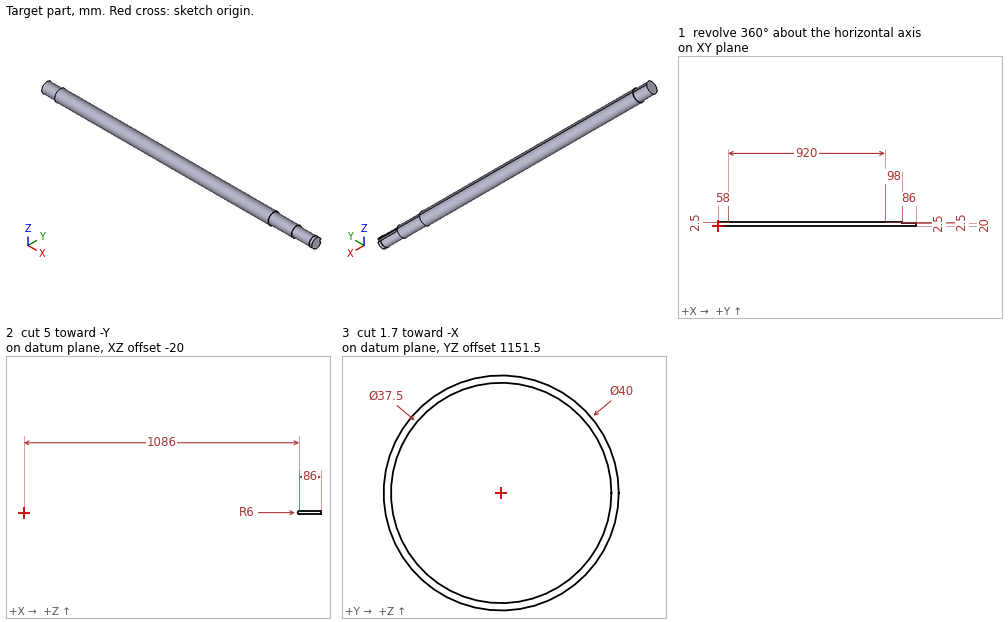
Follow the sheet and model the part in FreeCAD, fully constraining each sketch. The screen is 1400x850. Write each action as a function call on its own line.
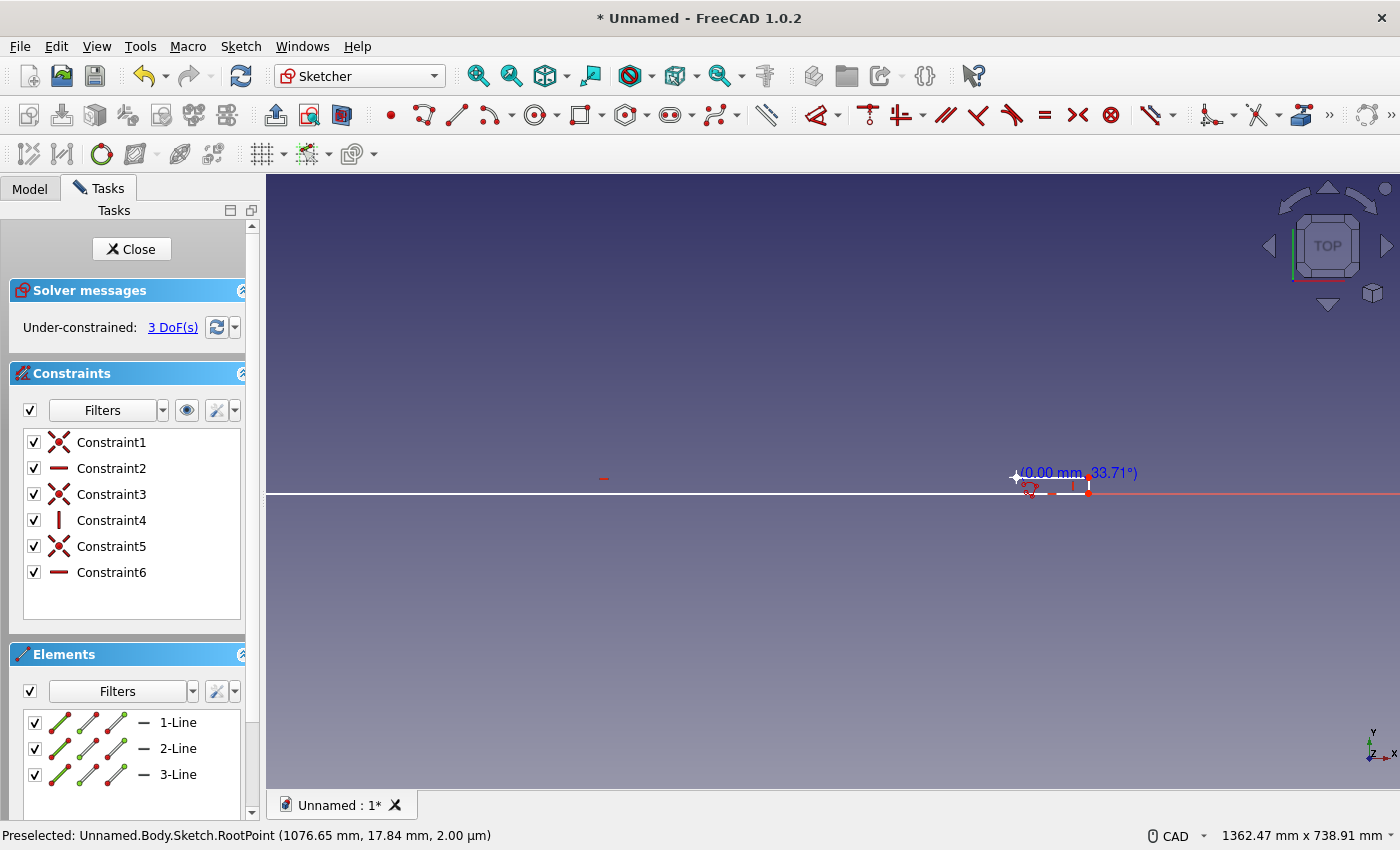
scroll(1016, 475, up, 11)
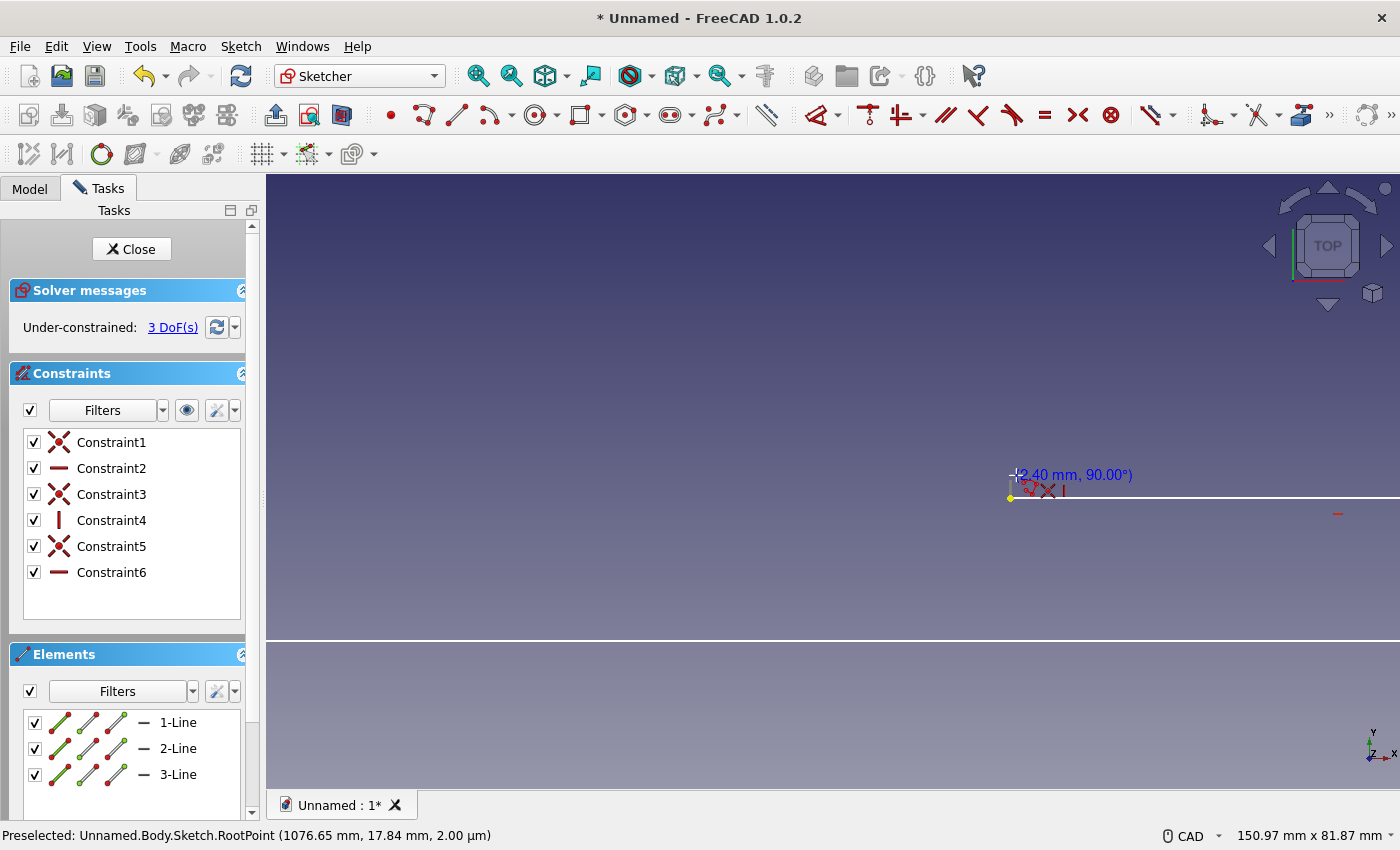
click(1011, 472)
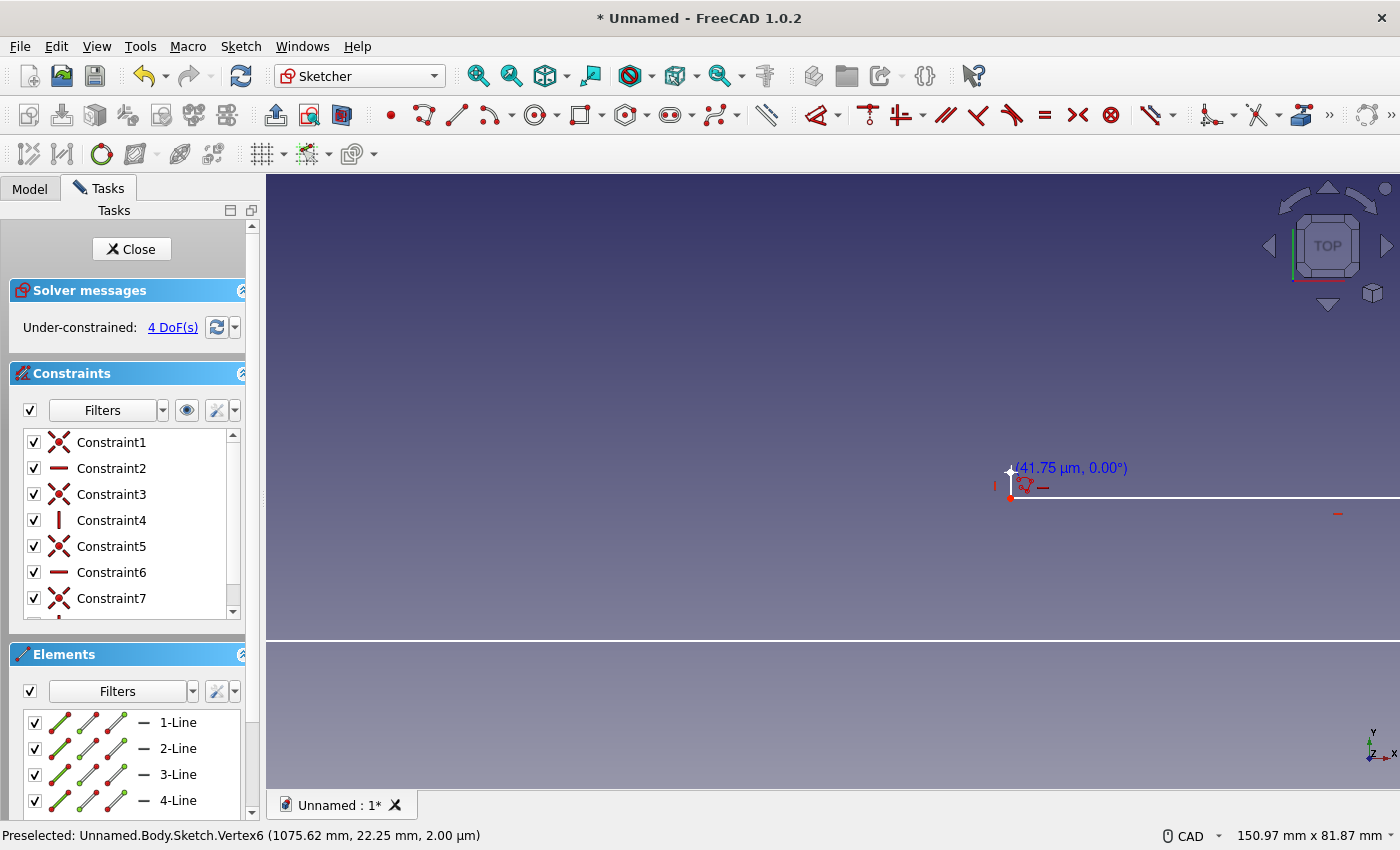
scroll(1043, 476, down, 13)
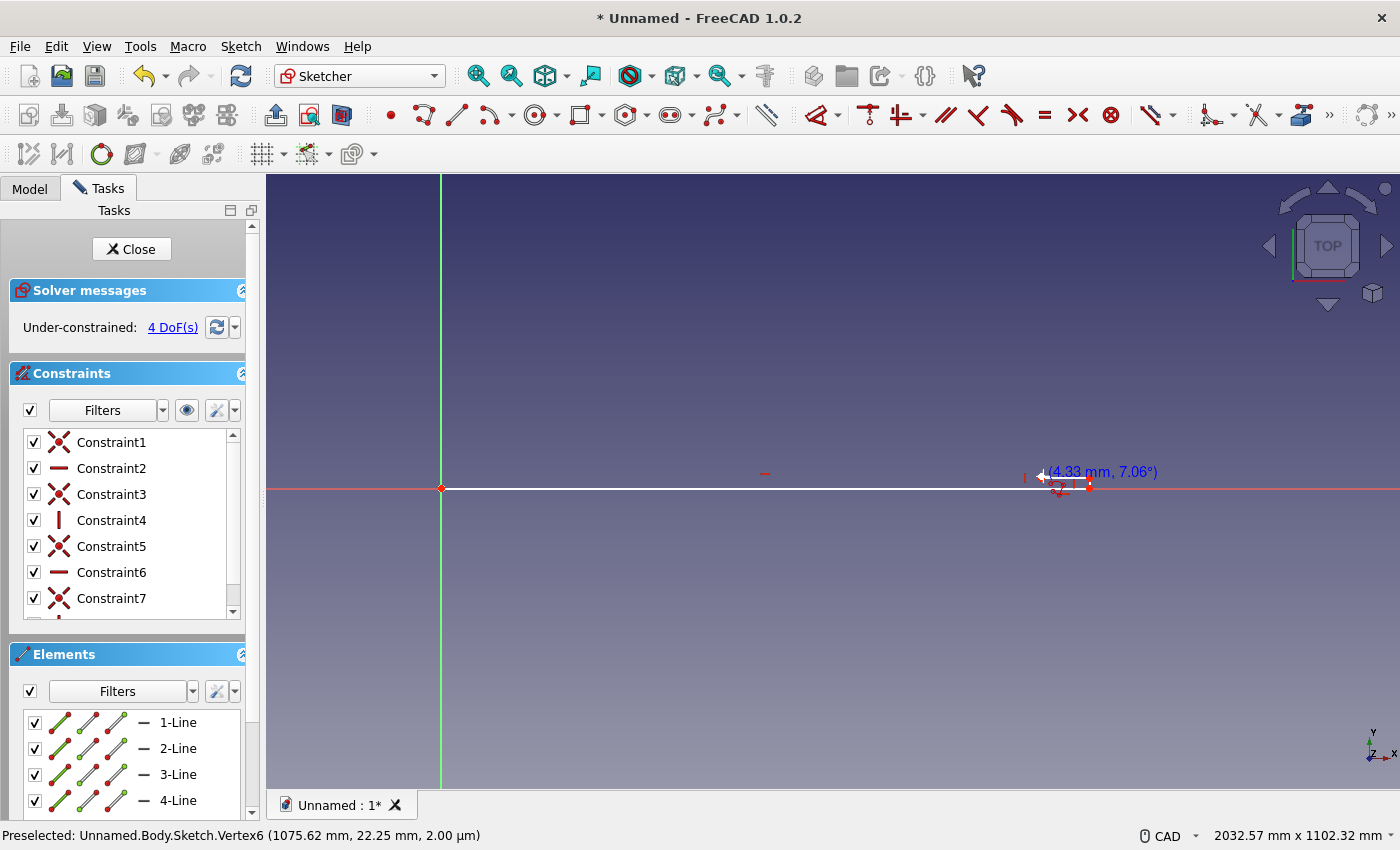
scroll(987, 476, up, 2)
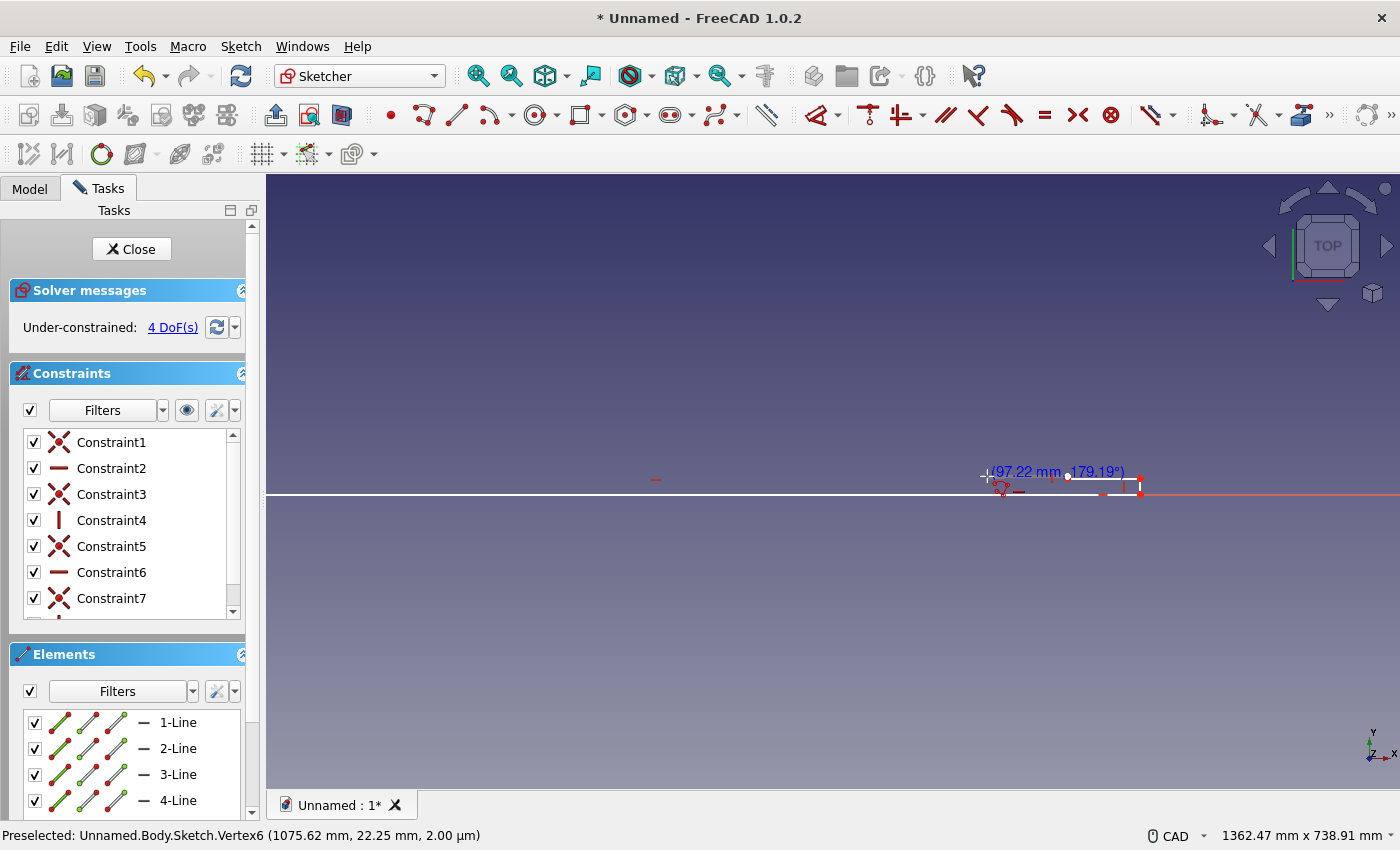
click(986, 476)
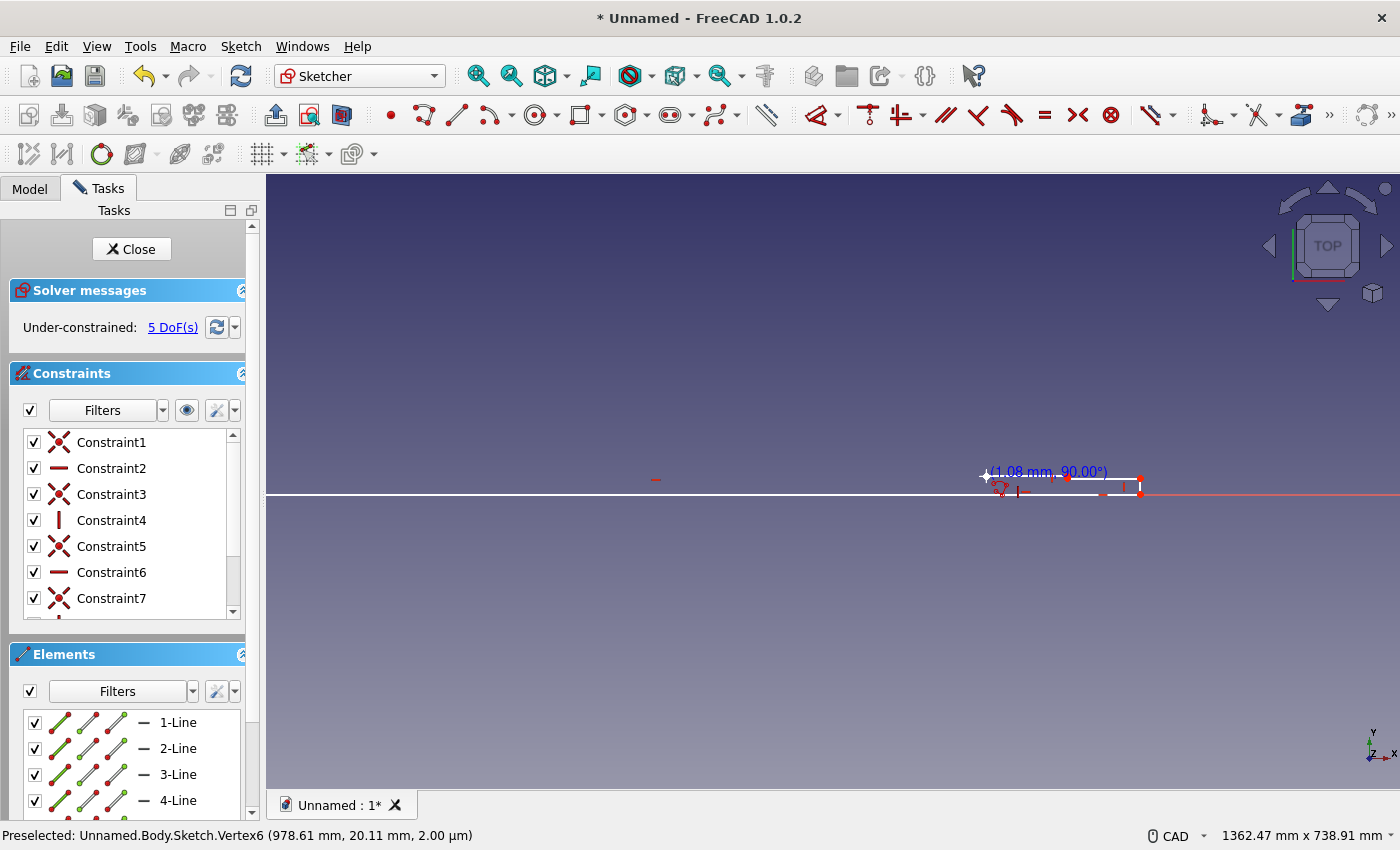
scroll(986, 474, up, 11)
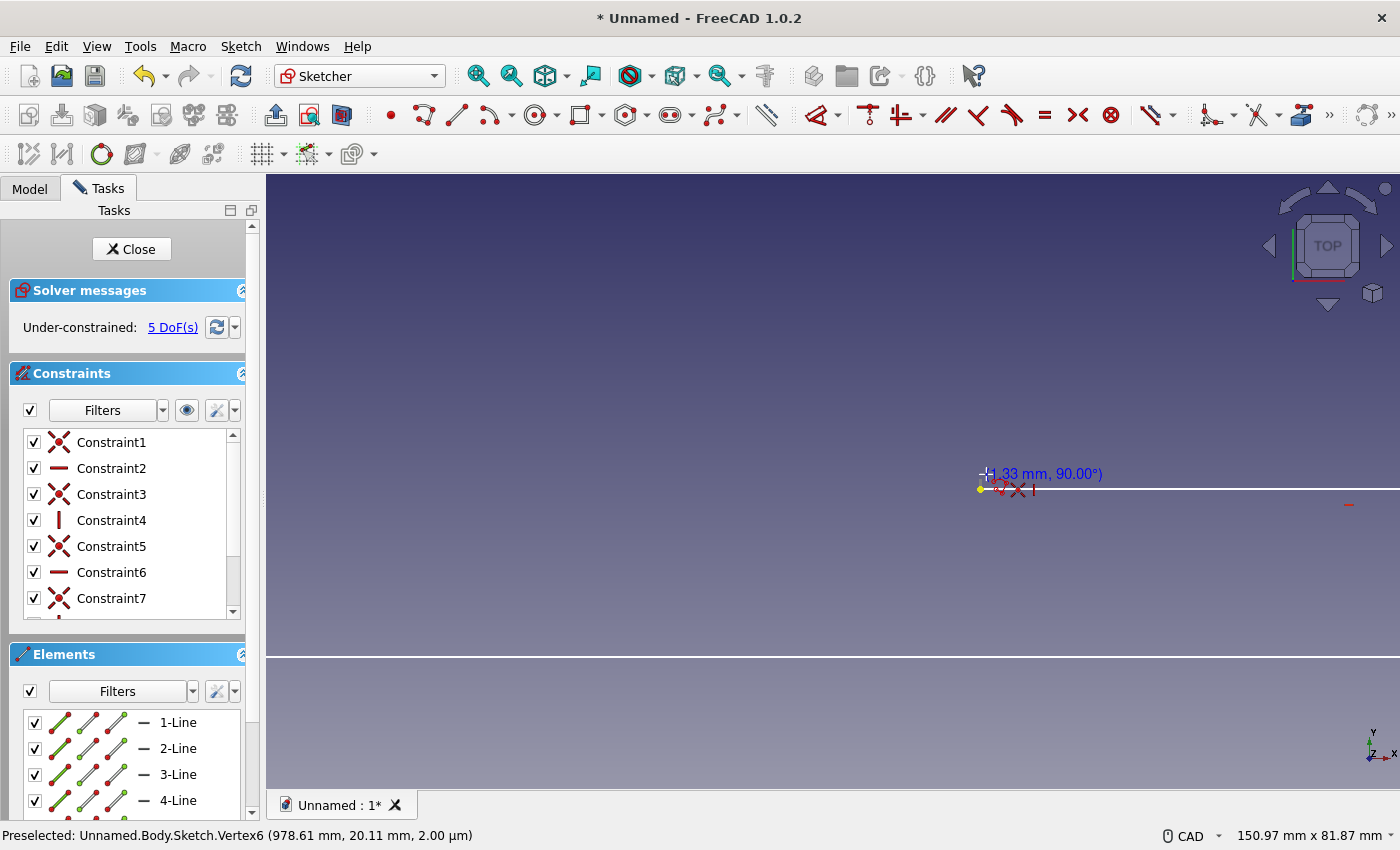
click(981, 469)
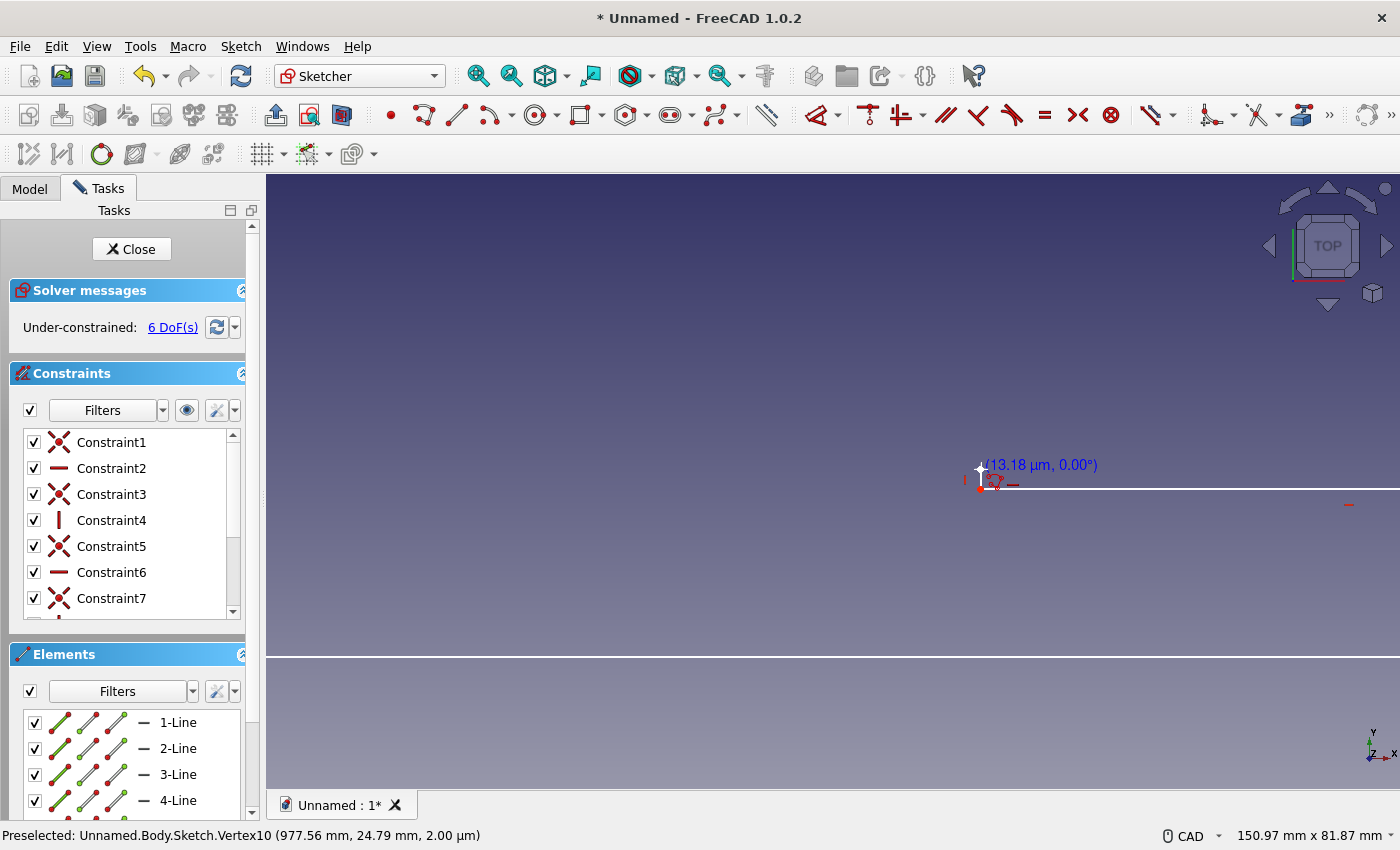
scroll(986, 475, down, 13)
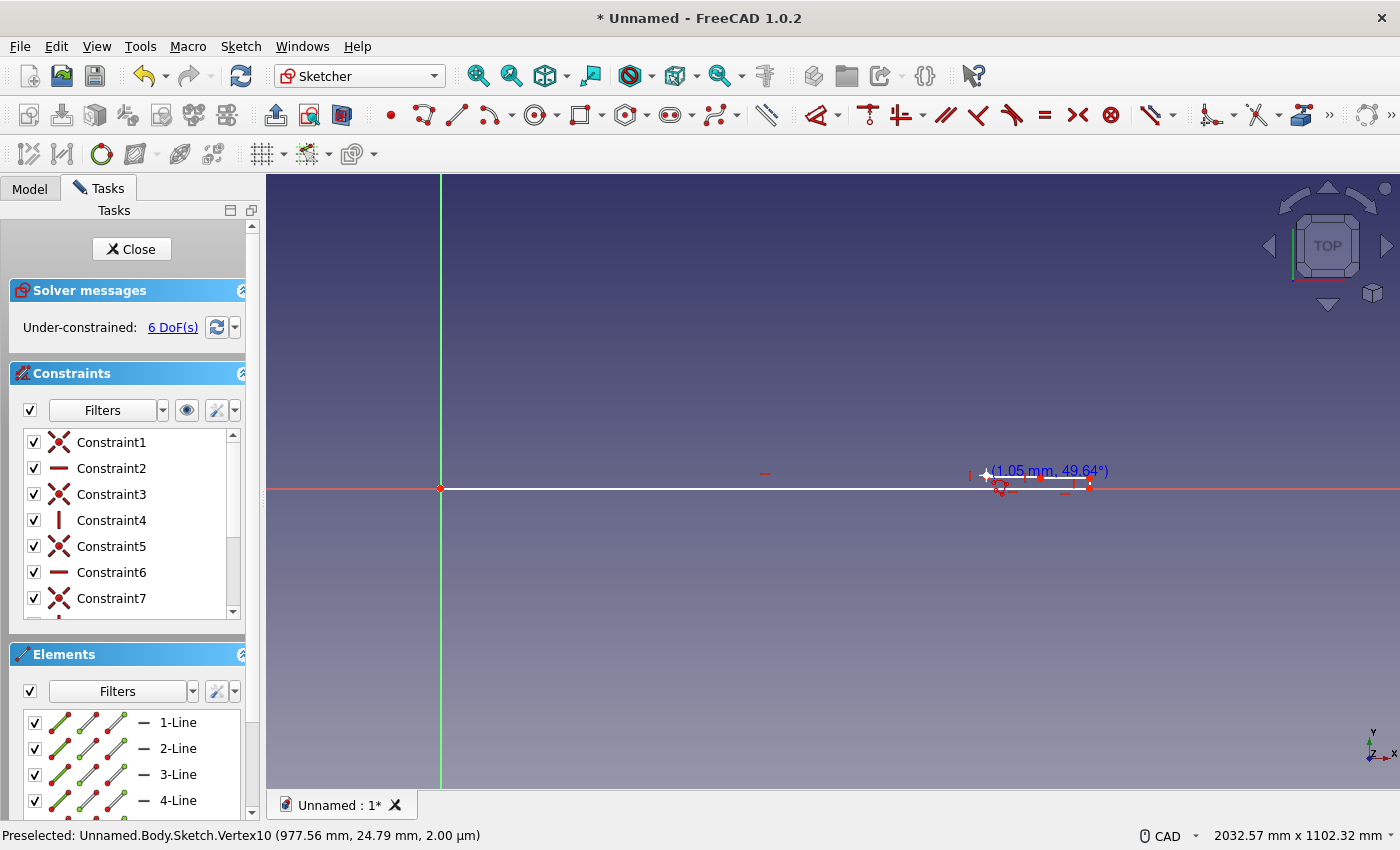
click(473, 475)